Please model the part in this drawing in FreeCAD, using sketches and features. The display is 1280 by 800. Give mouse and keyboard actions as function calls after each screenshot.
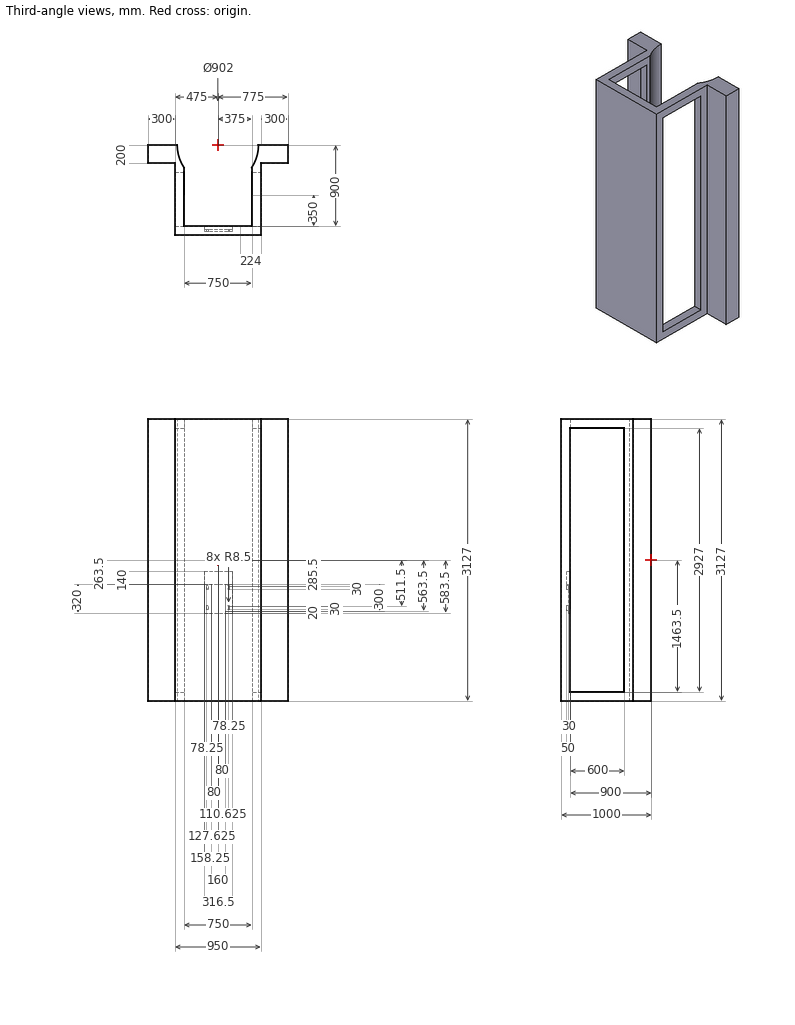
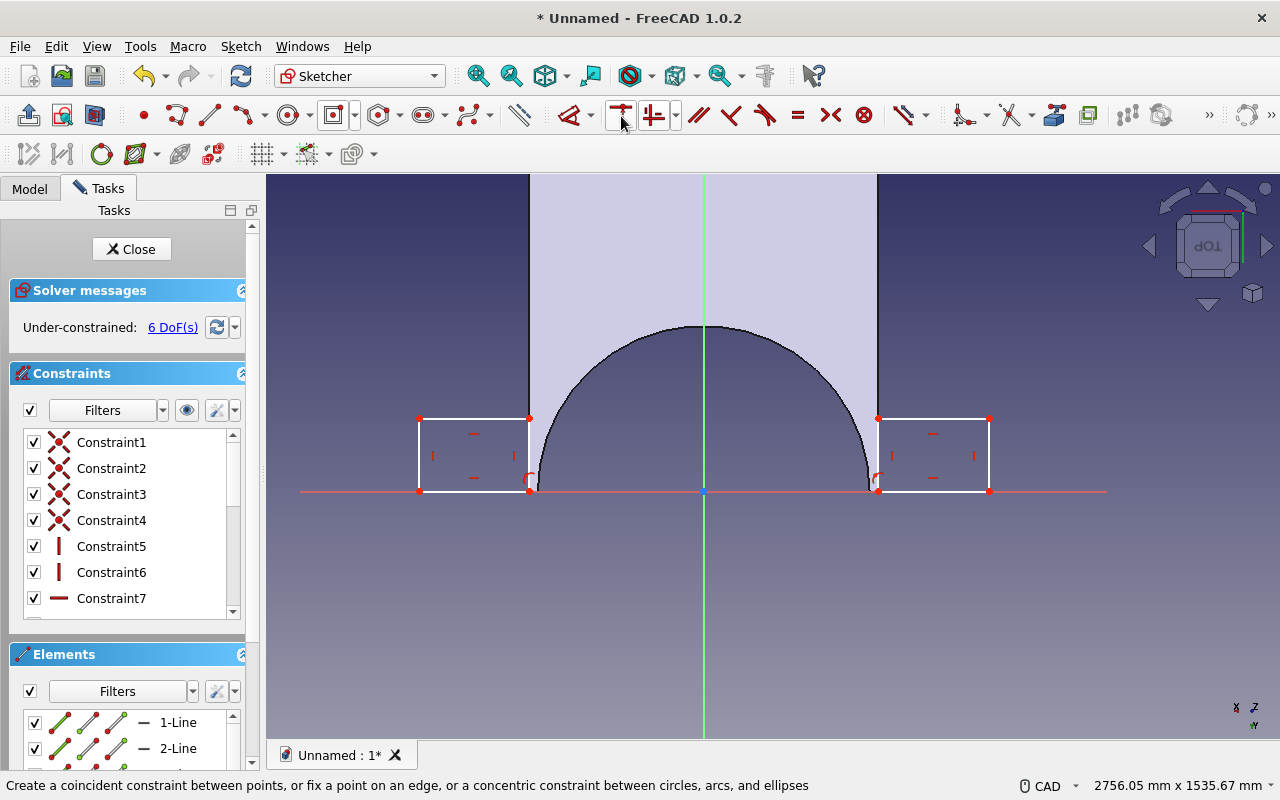
click(568, 116)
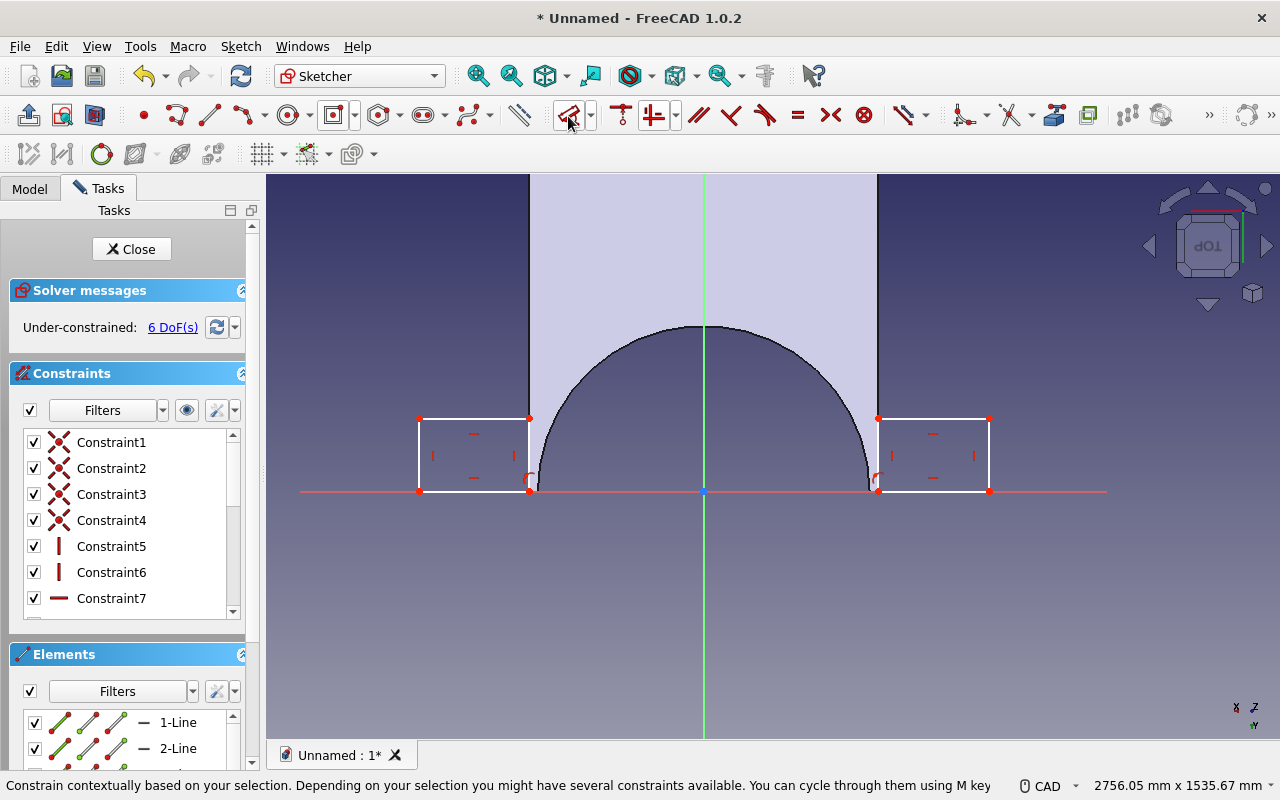
click(878, 441)
click(912, 455)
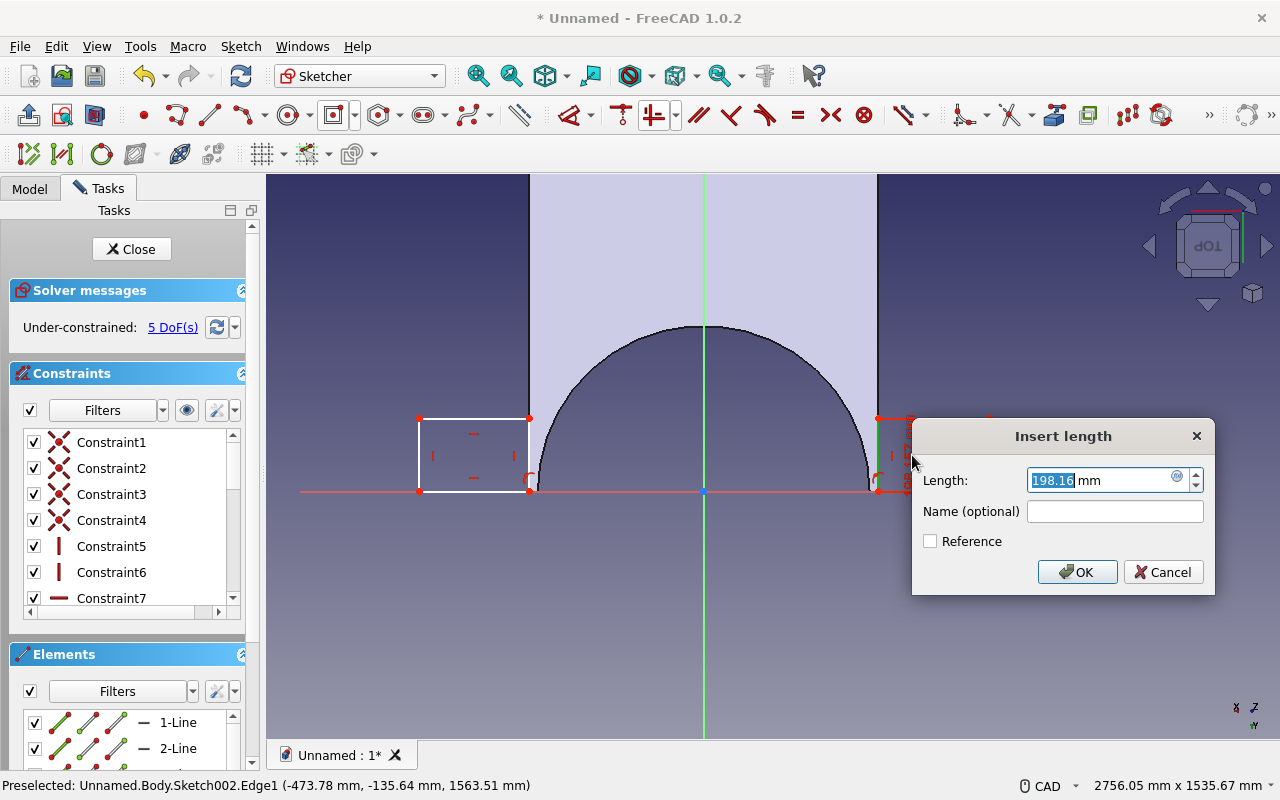
text(200)
key(Return)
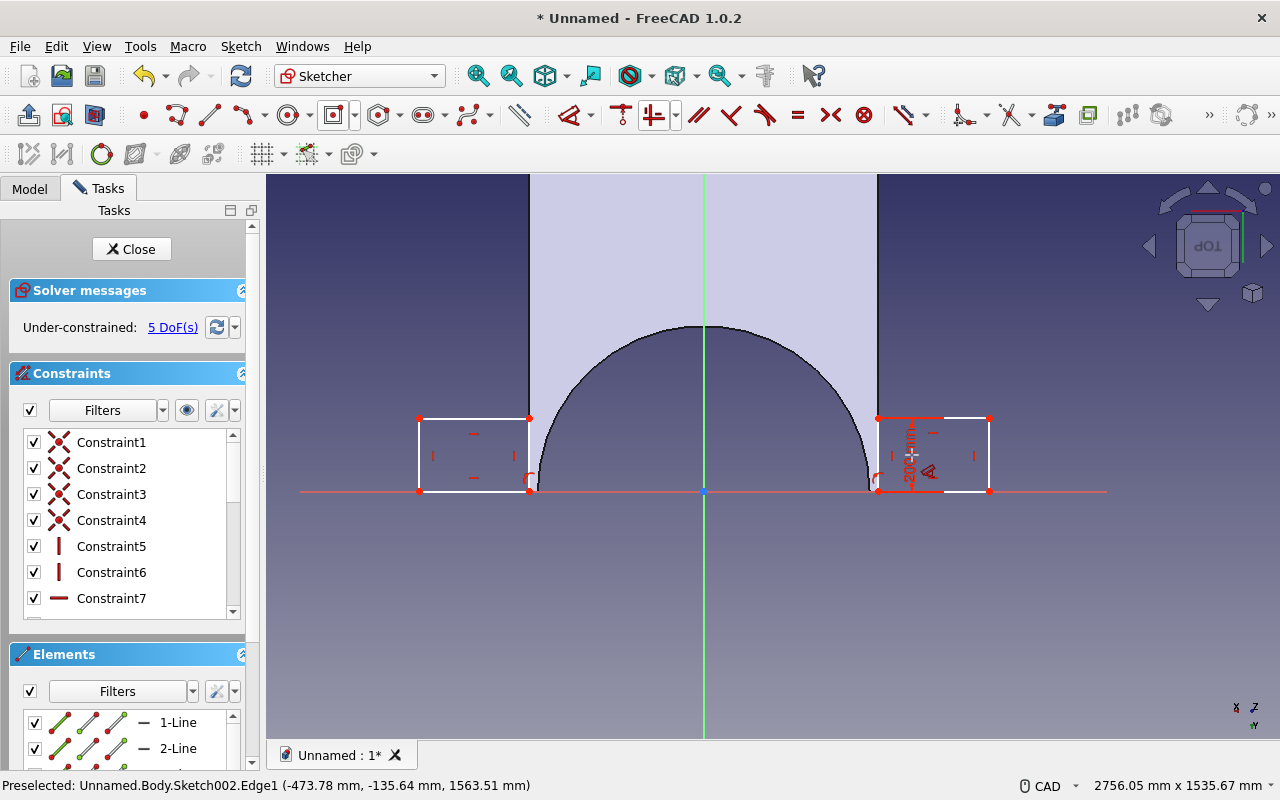
click(911, 492)
click(934, 526)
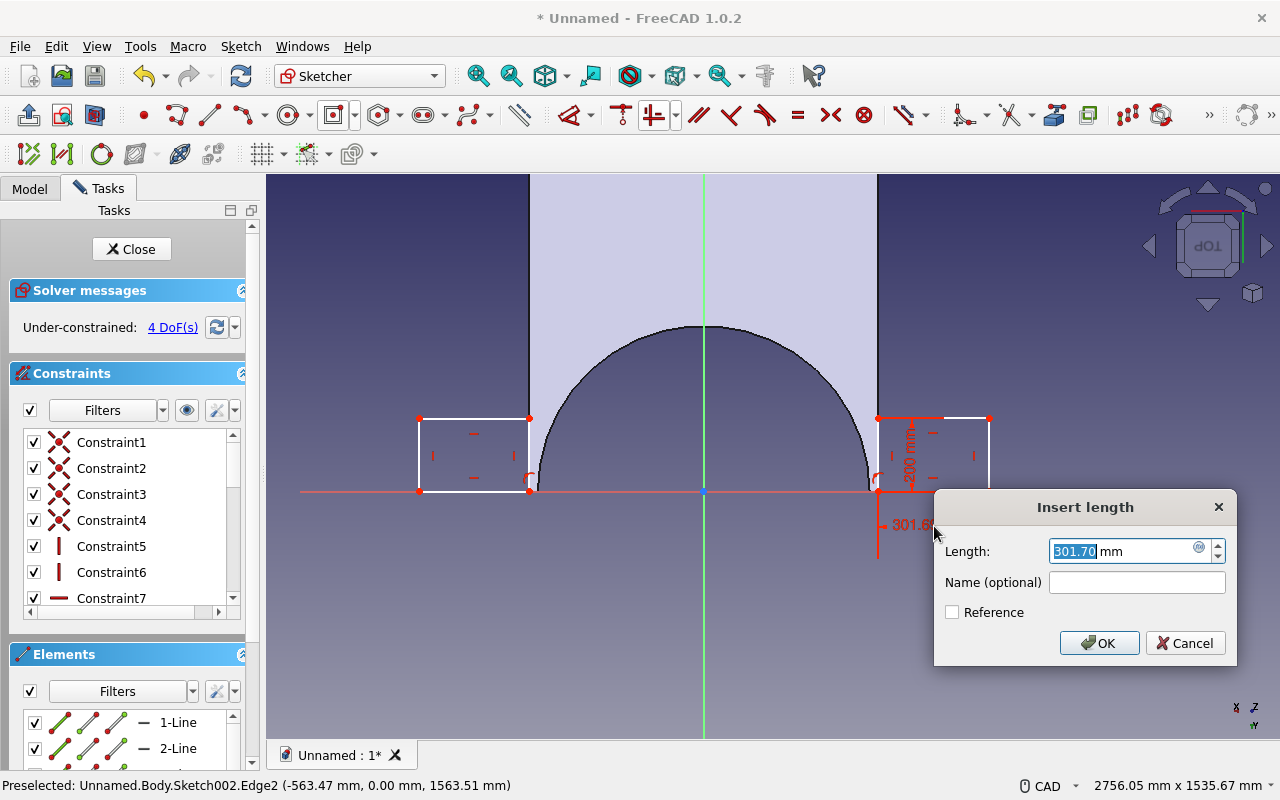
text(300)
key(Return)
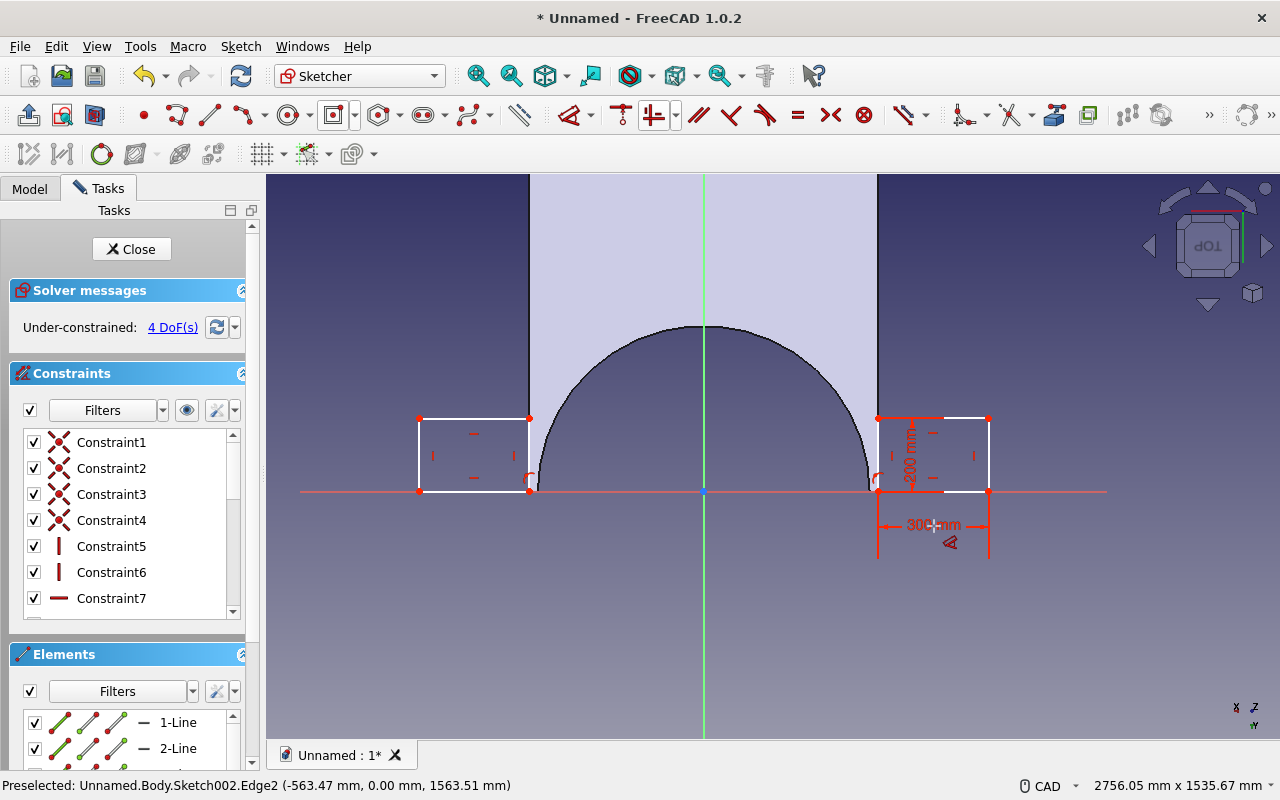
click(419, 441)
click(385, 455)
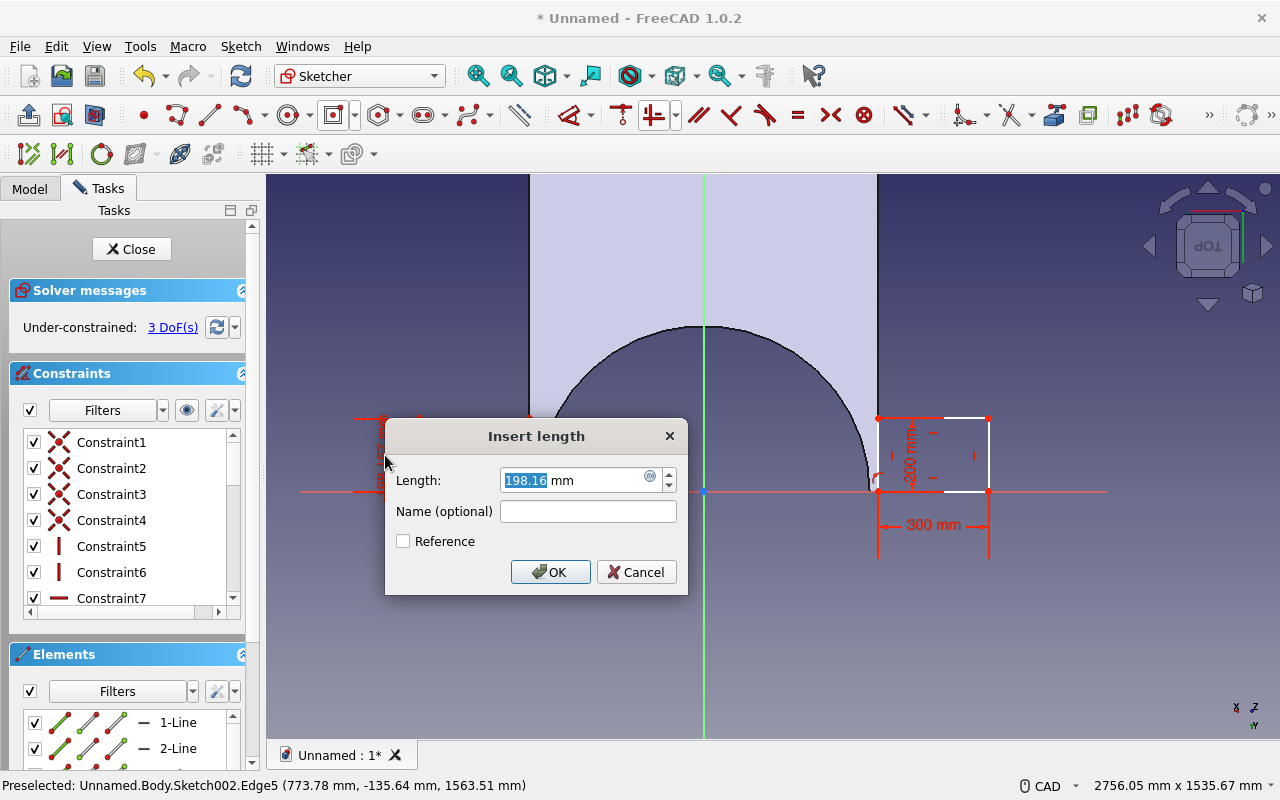
text(200)
key(Return)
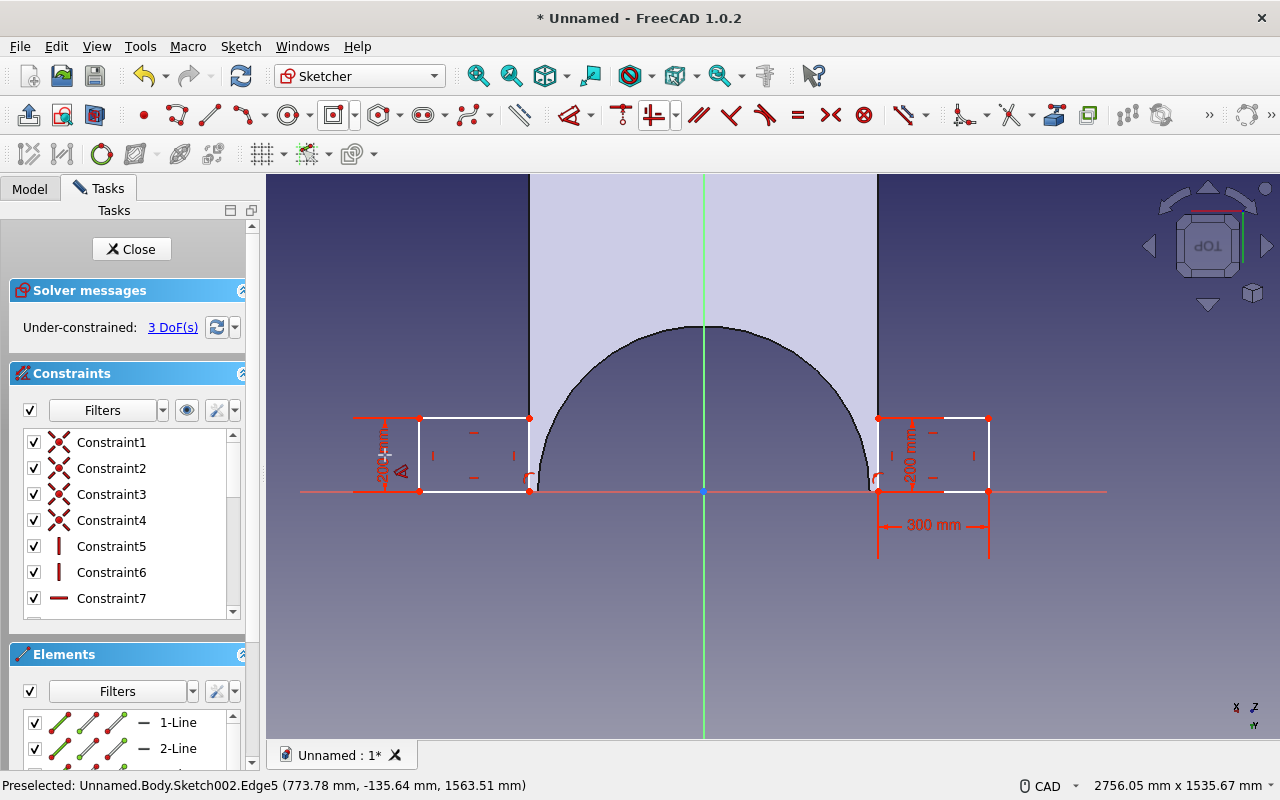
click(452, 492)
click(474, 526)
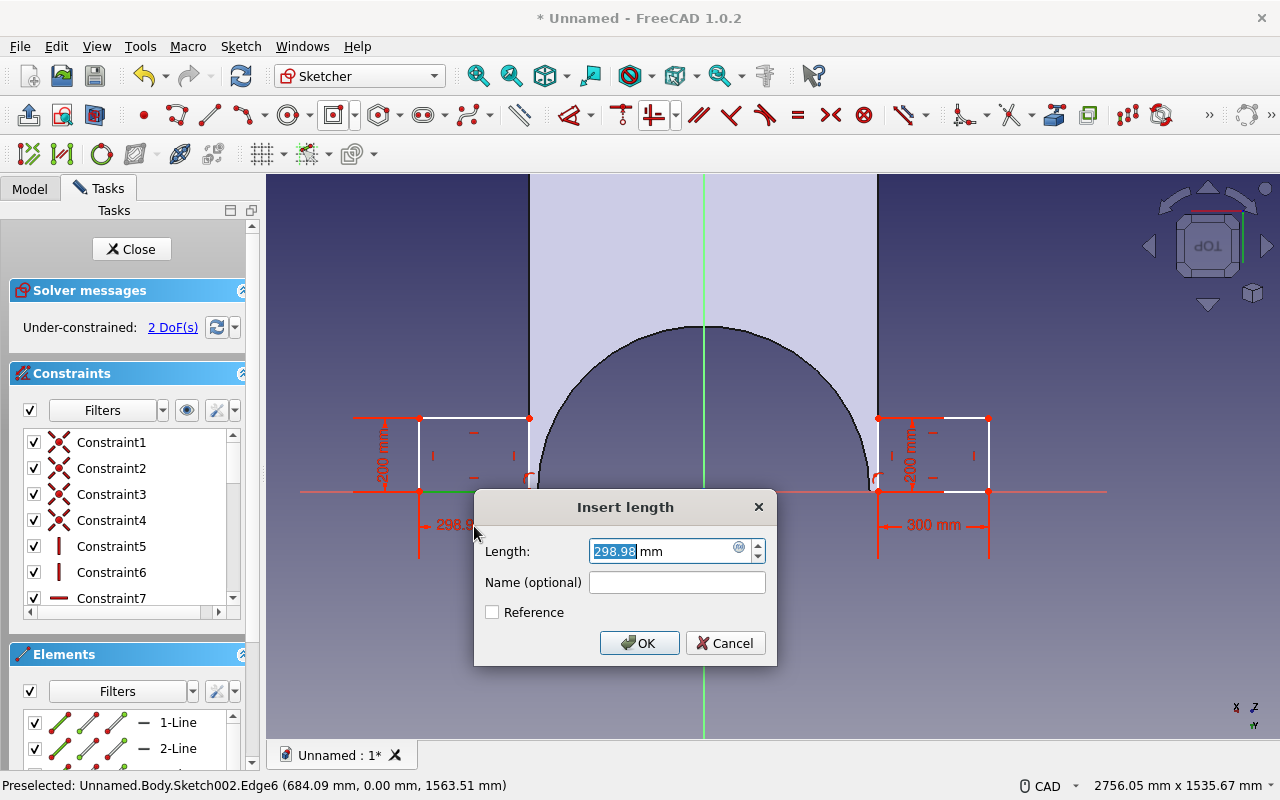
text(300)
key(Return)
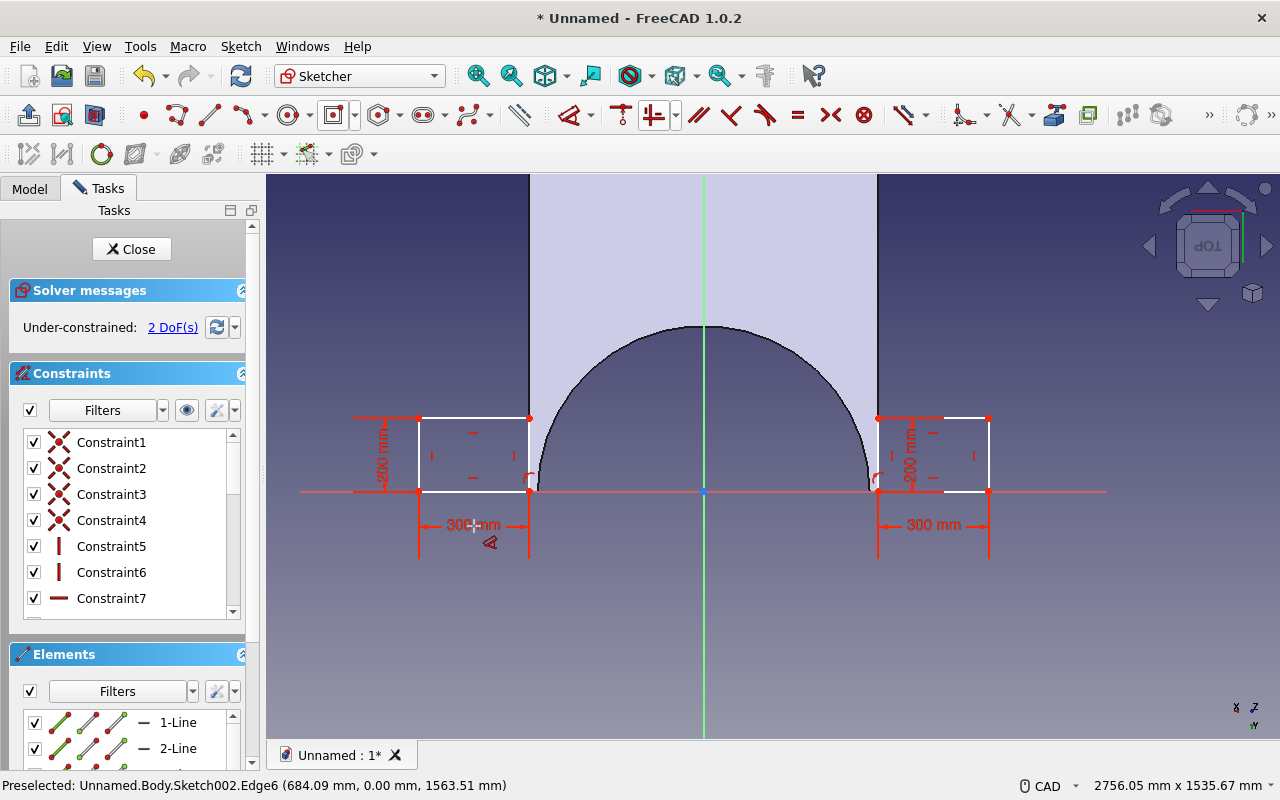
click(878, 418)
click(791, 526)